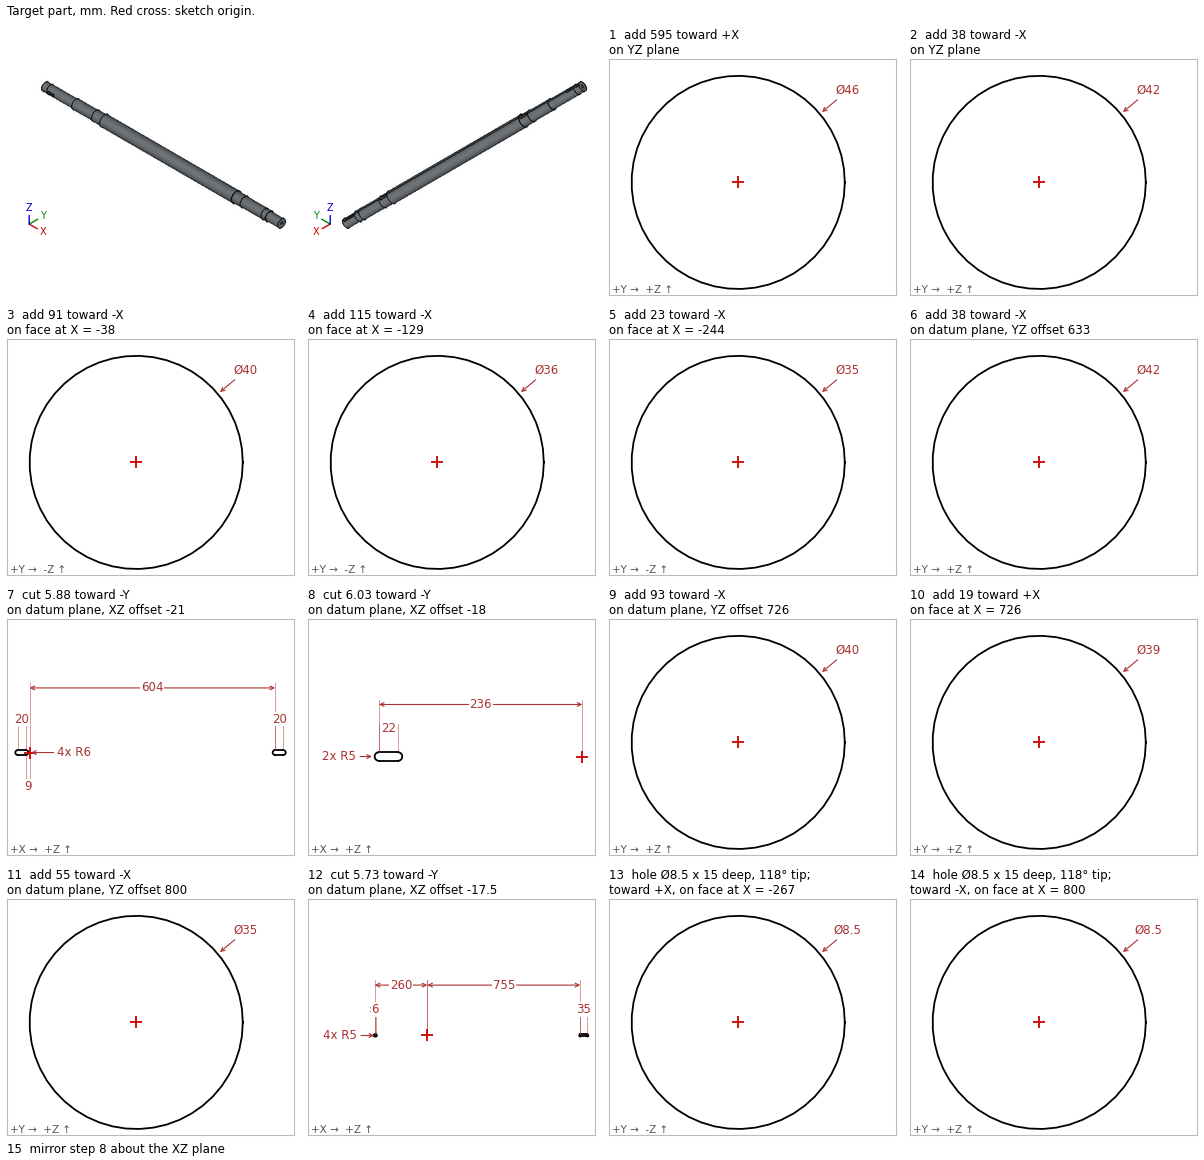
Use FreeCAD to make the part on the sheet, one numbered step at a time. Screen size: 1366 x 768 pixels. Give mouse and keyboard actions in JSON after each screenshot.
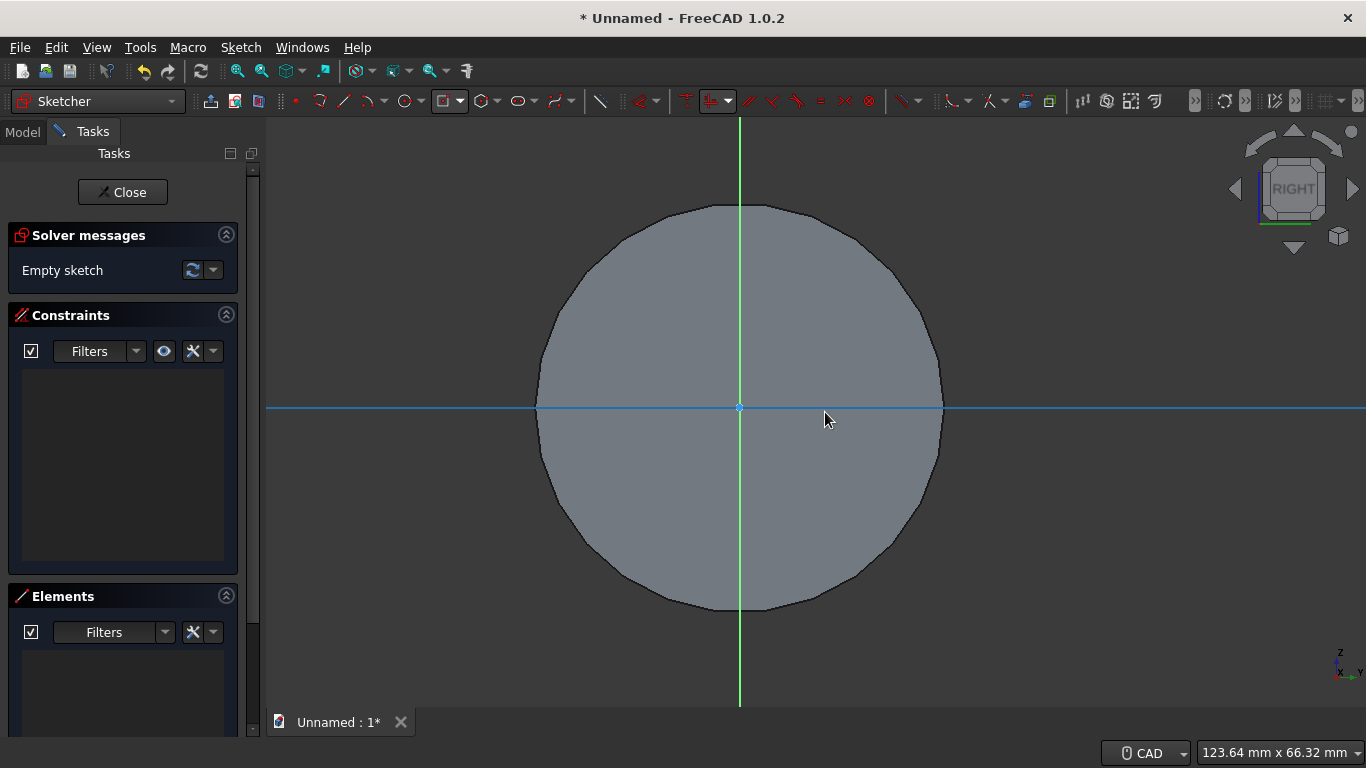
{"action": "key", "text": "g c"}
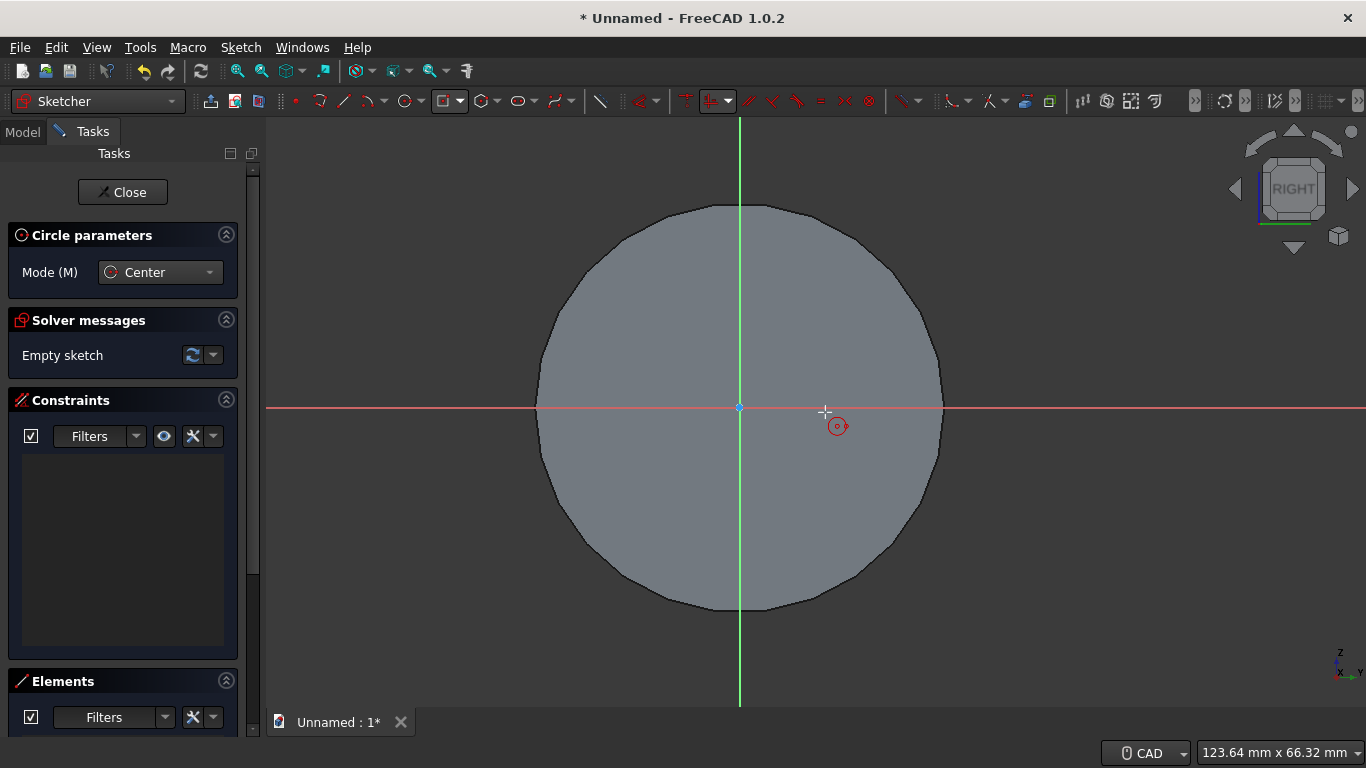
{"action": "left_click", "coordinate": [740, 408]}
{"action": "mouse_move", "coordinate": [872, 276]}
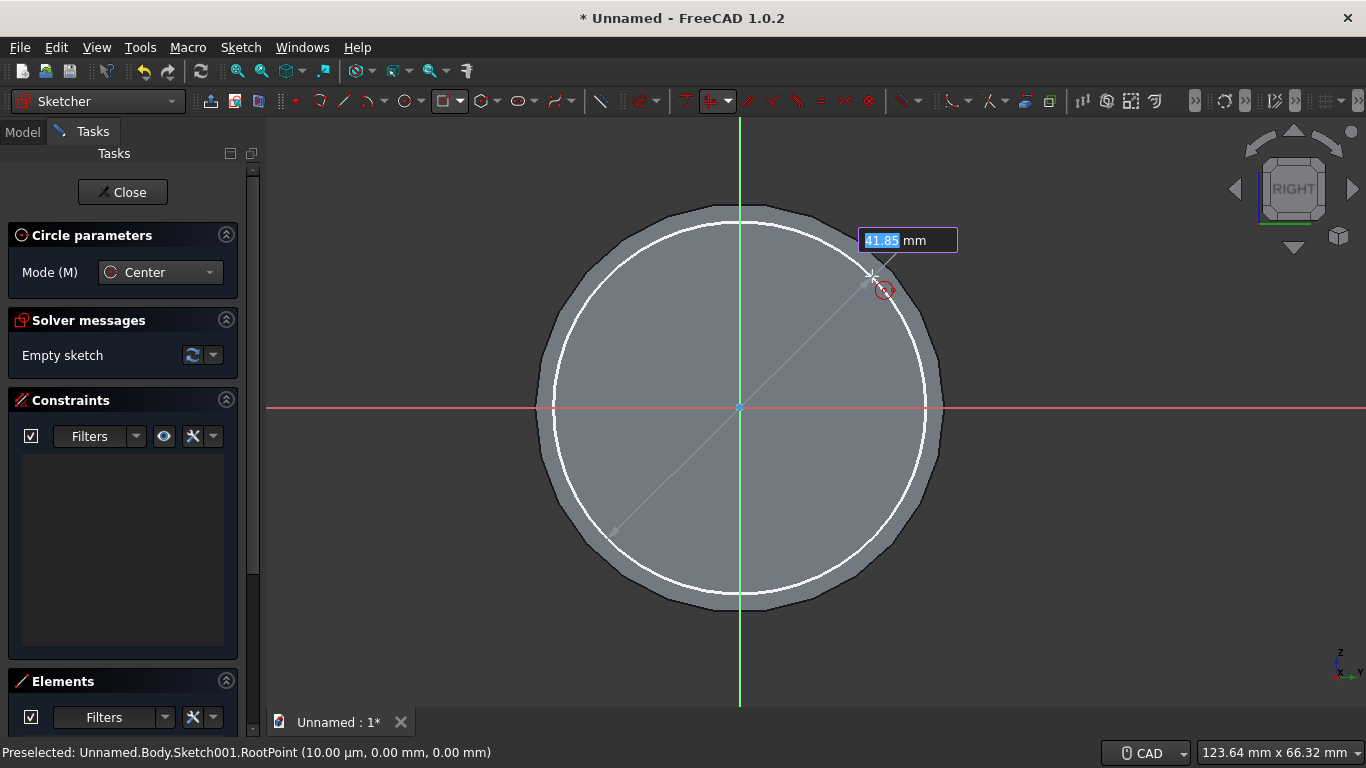
{"action": "type", "text": "42"}
{"action": "key", "text": "Return"}
{"action": "key", "text": "Escape"}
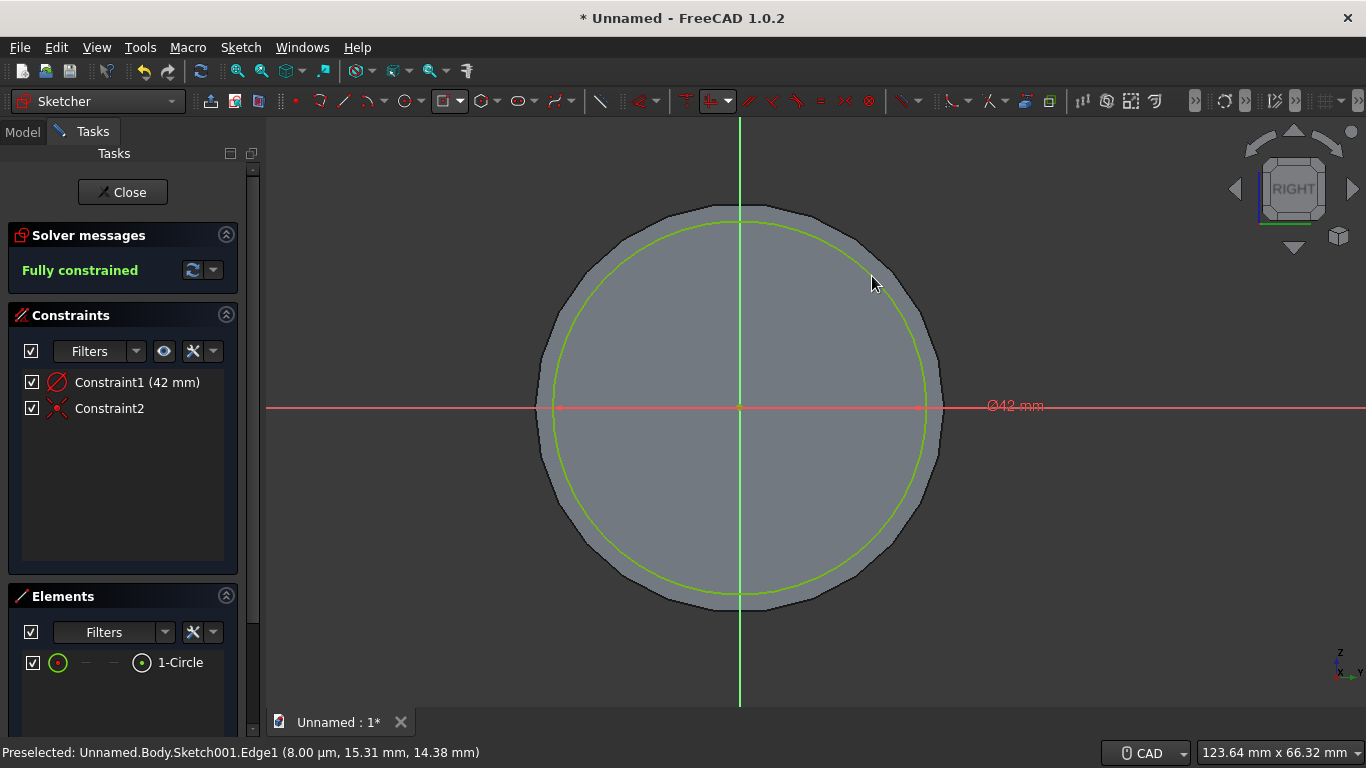
{"action": "left_click", "coordinate": [123, 192]}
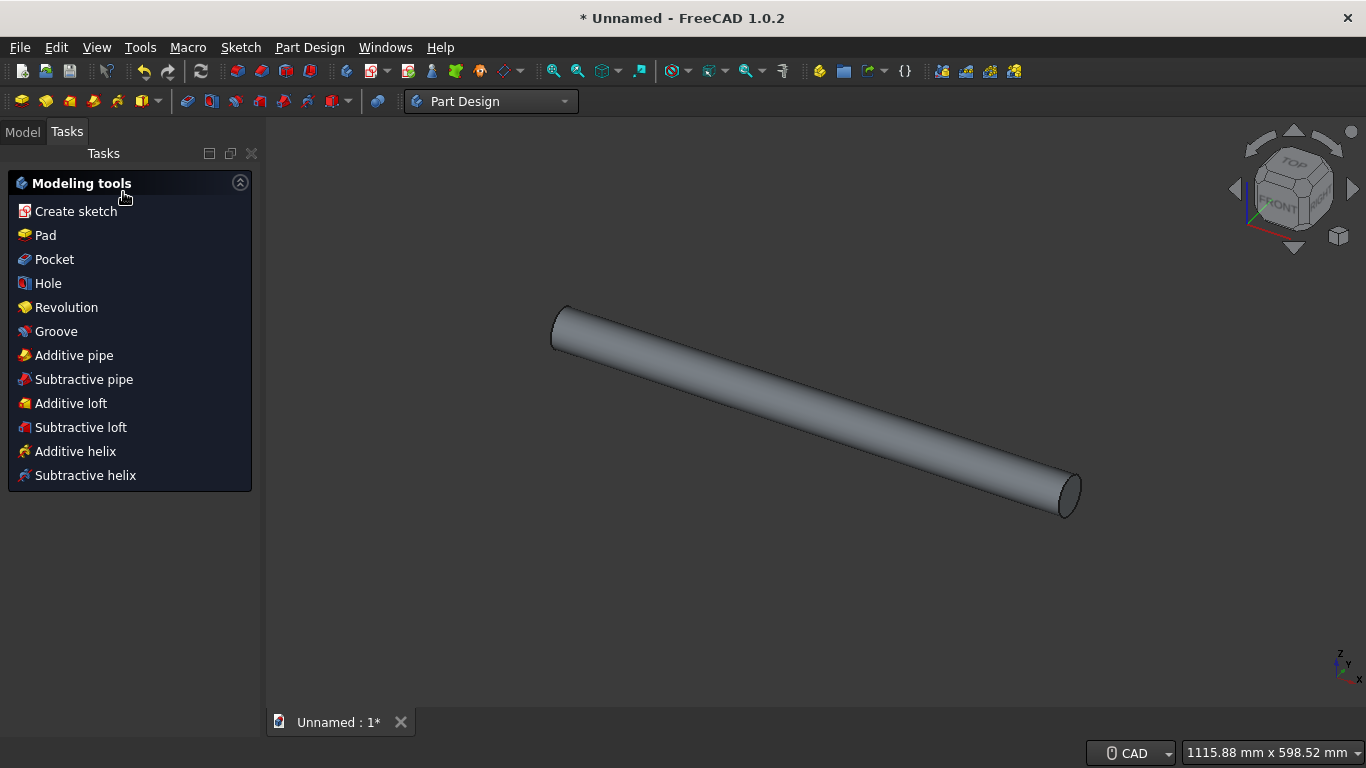
{"action": "left_click", "coordinate": [22, 102]}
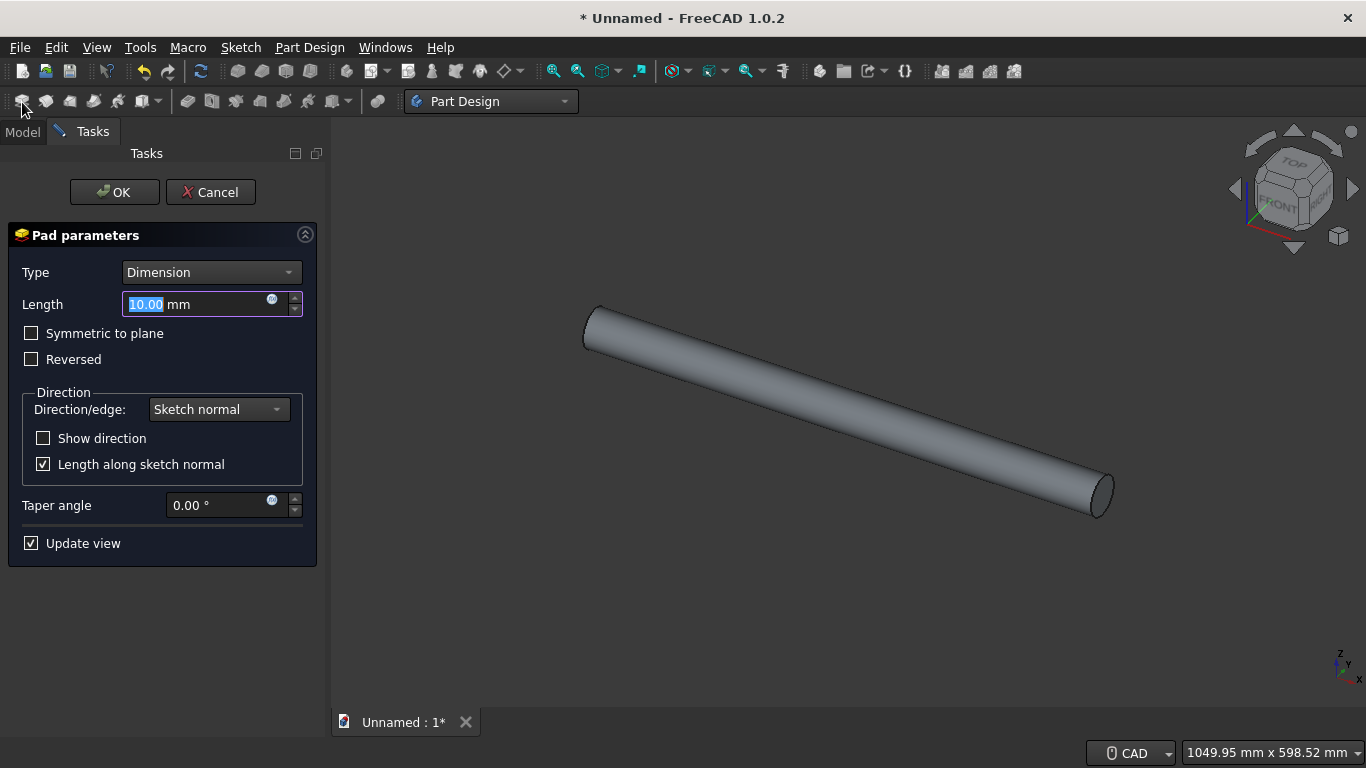
{"action": "type", "text": "38"}
{"action": "key", "text": "Tab"}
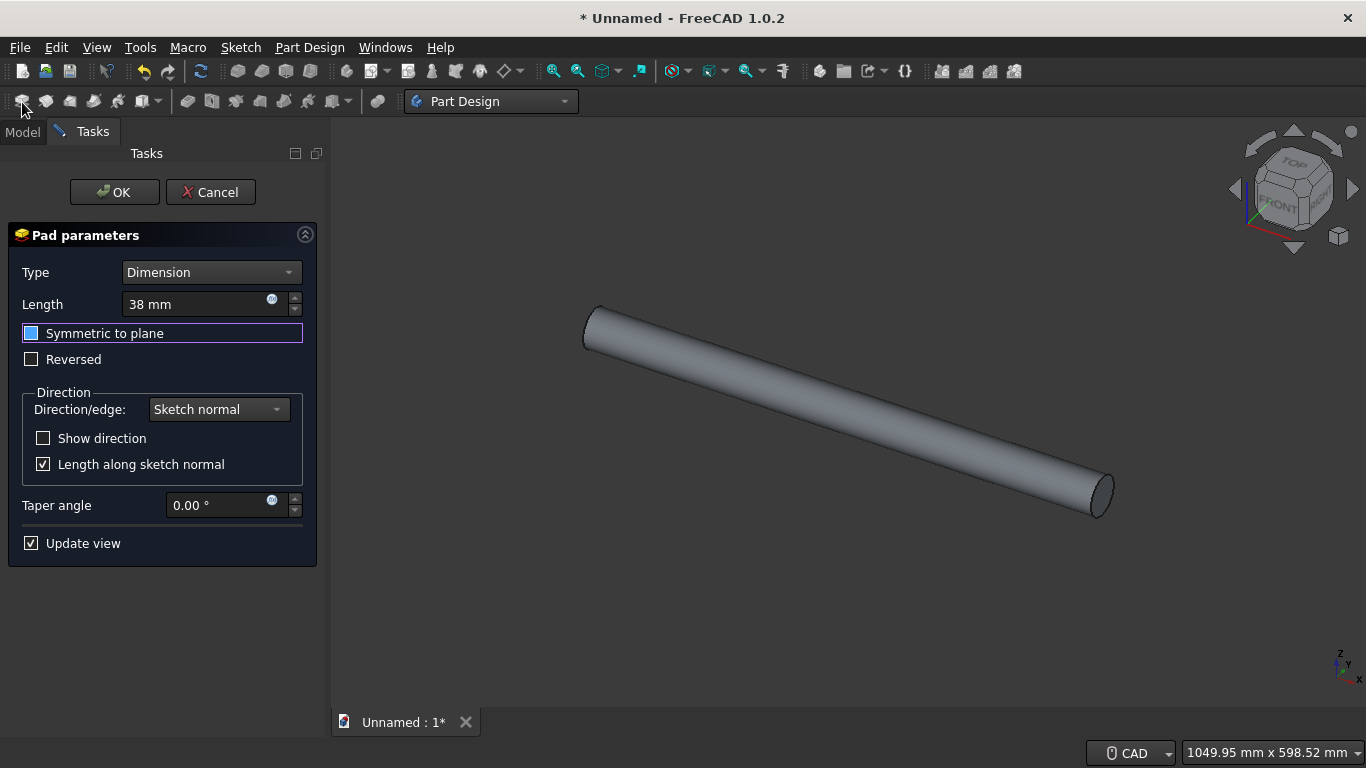
{"action": "left_click", "coordinate": [30, 359]}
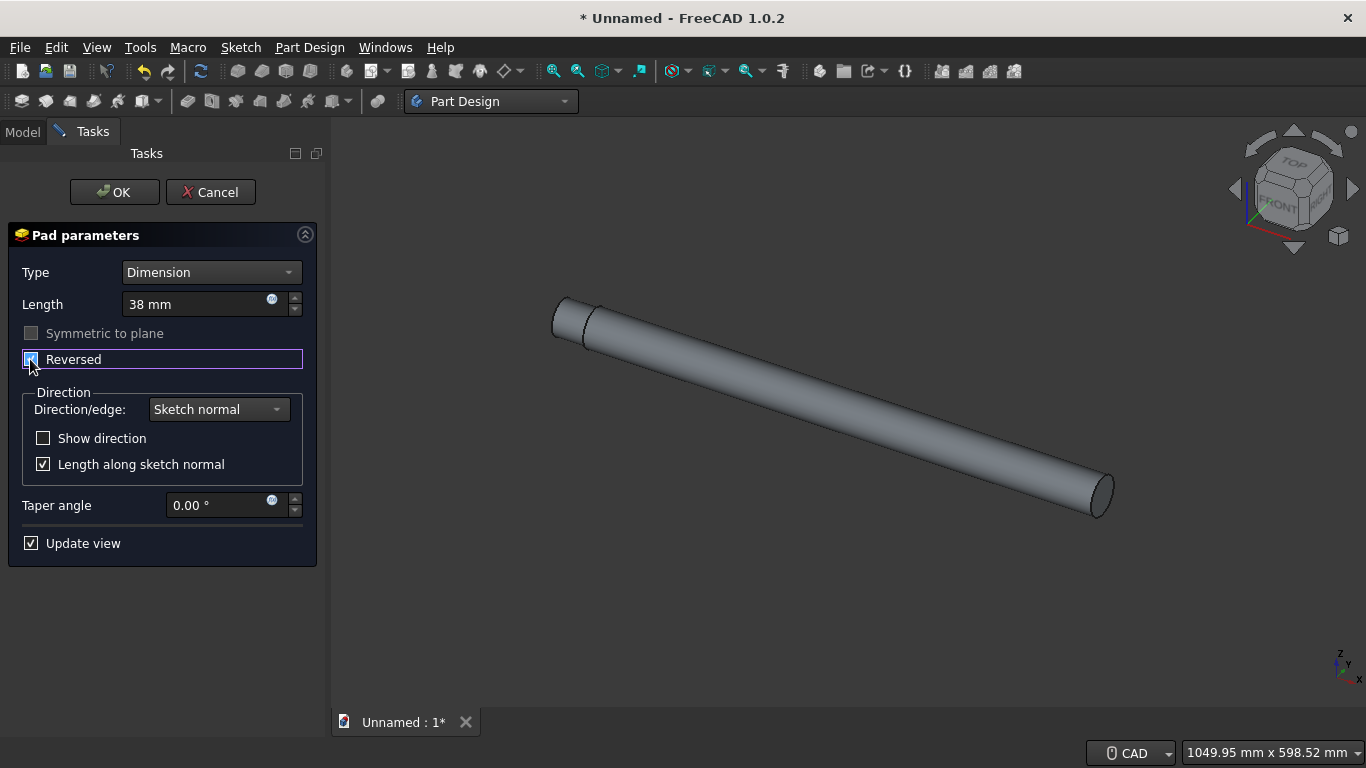
{"action": "left_click", "coordinate": [115, 192]}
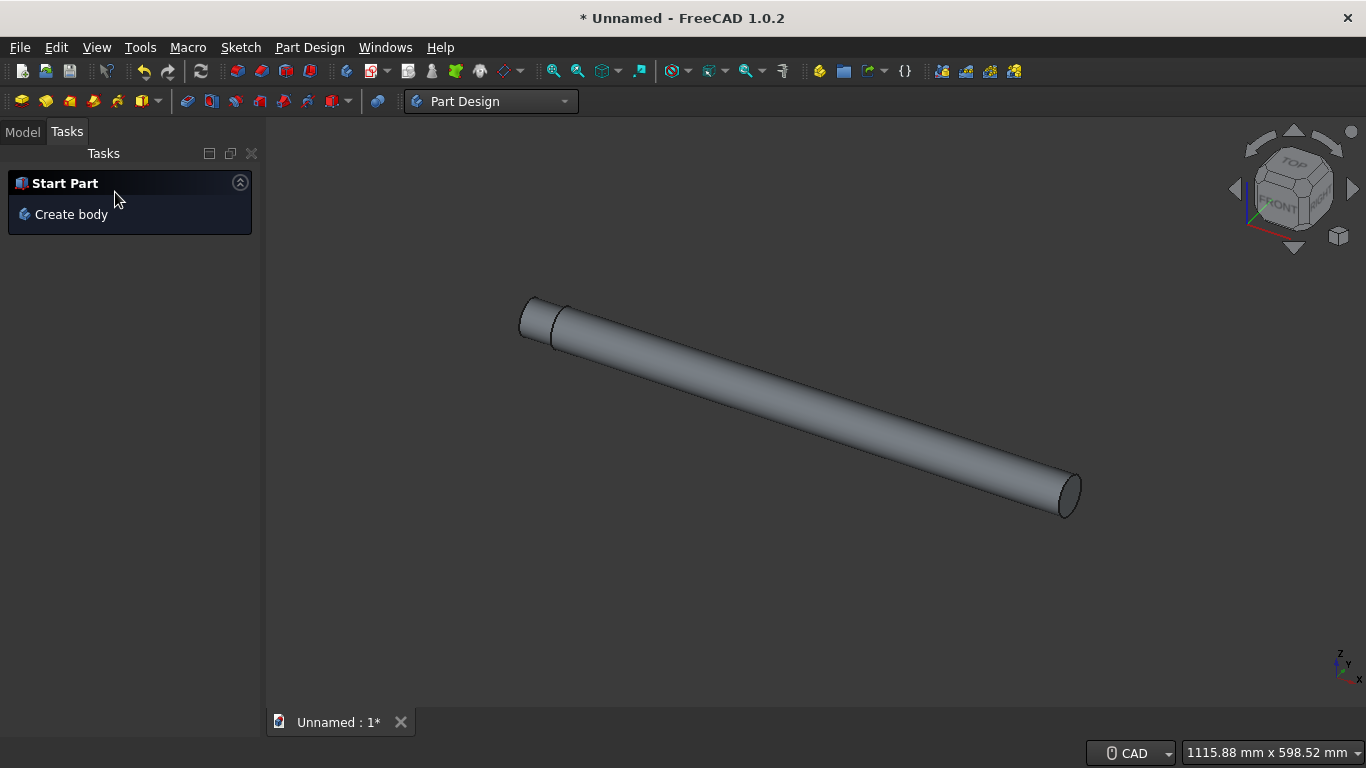
{"action": "key", "text": "6"}